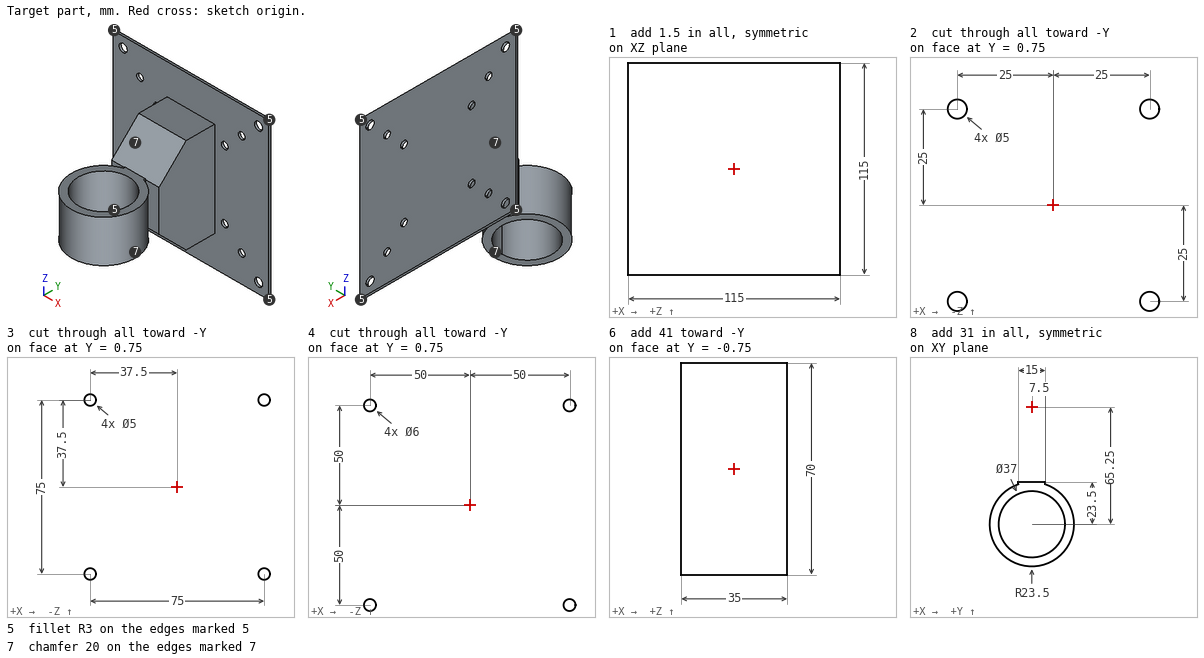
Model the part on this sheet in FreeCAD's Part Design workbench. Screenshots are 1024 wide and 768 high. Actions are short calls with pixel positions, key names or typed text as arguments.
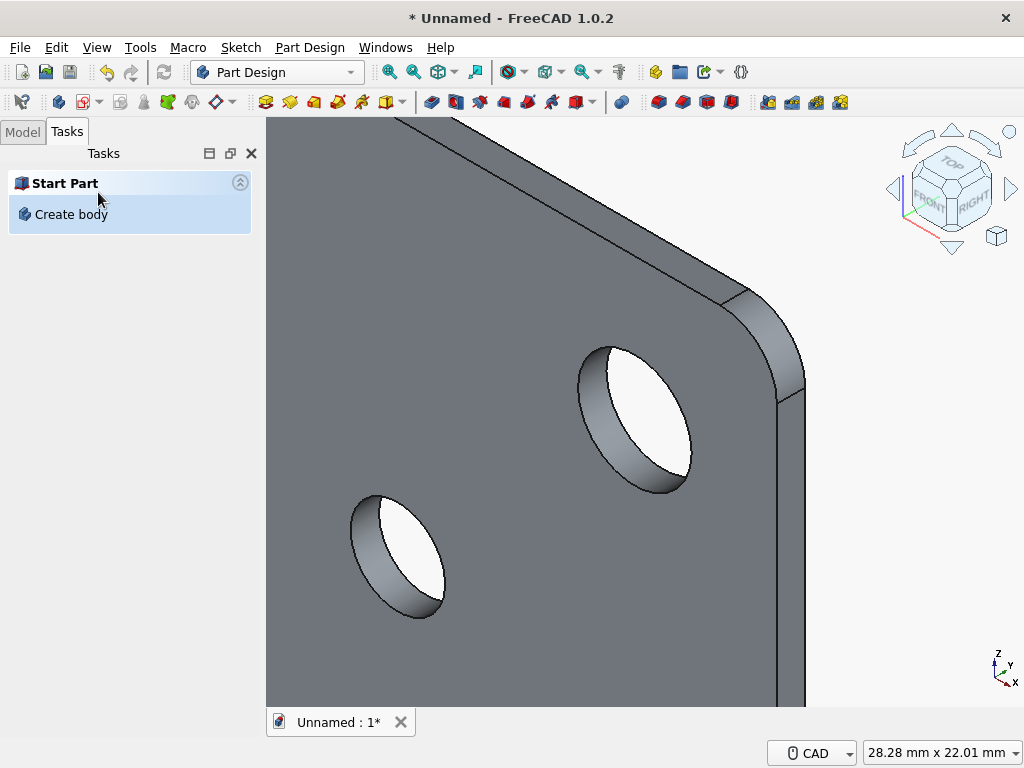
key(v)
key(f)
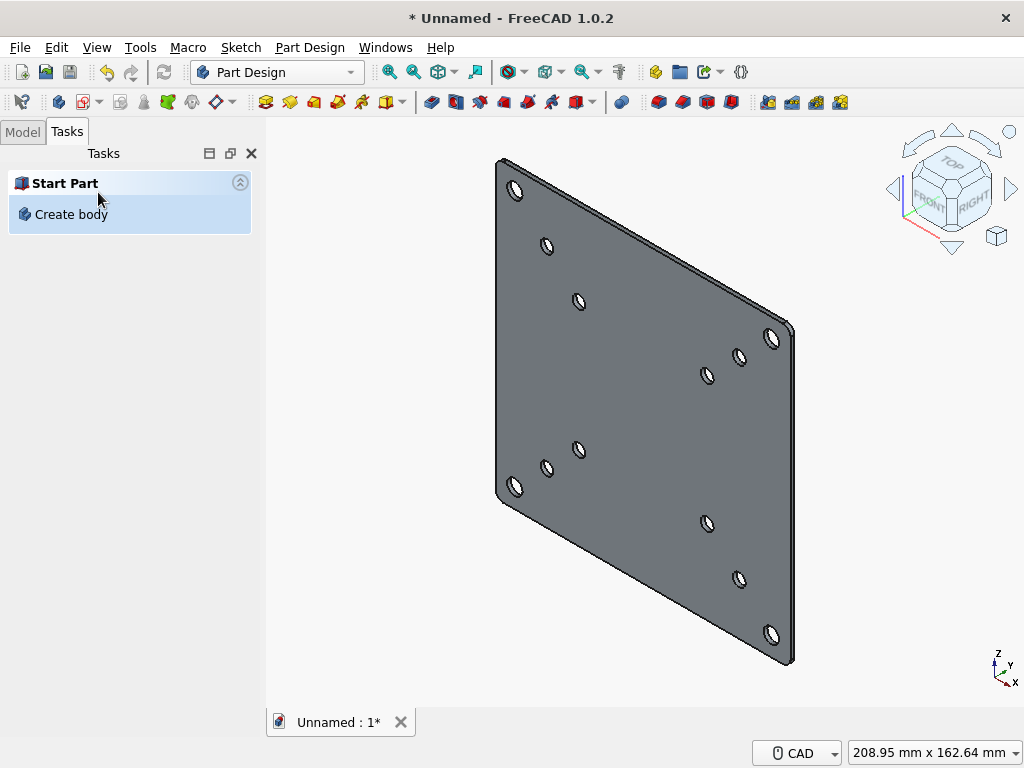
click(643, 412)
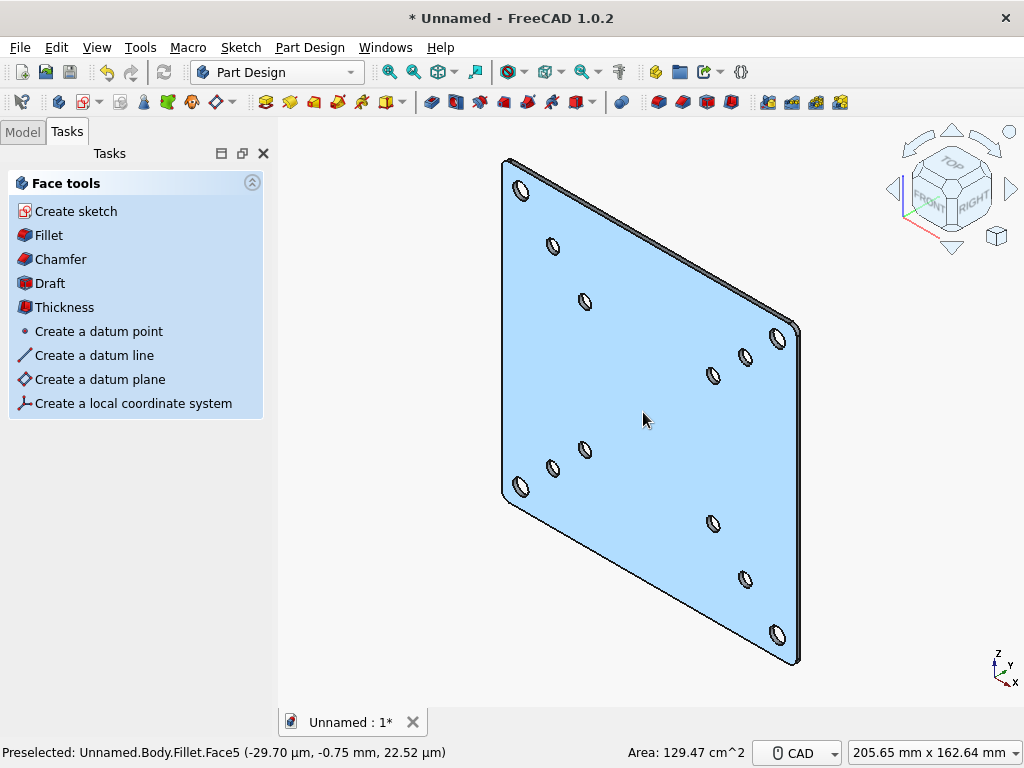
click(84, 102)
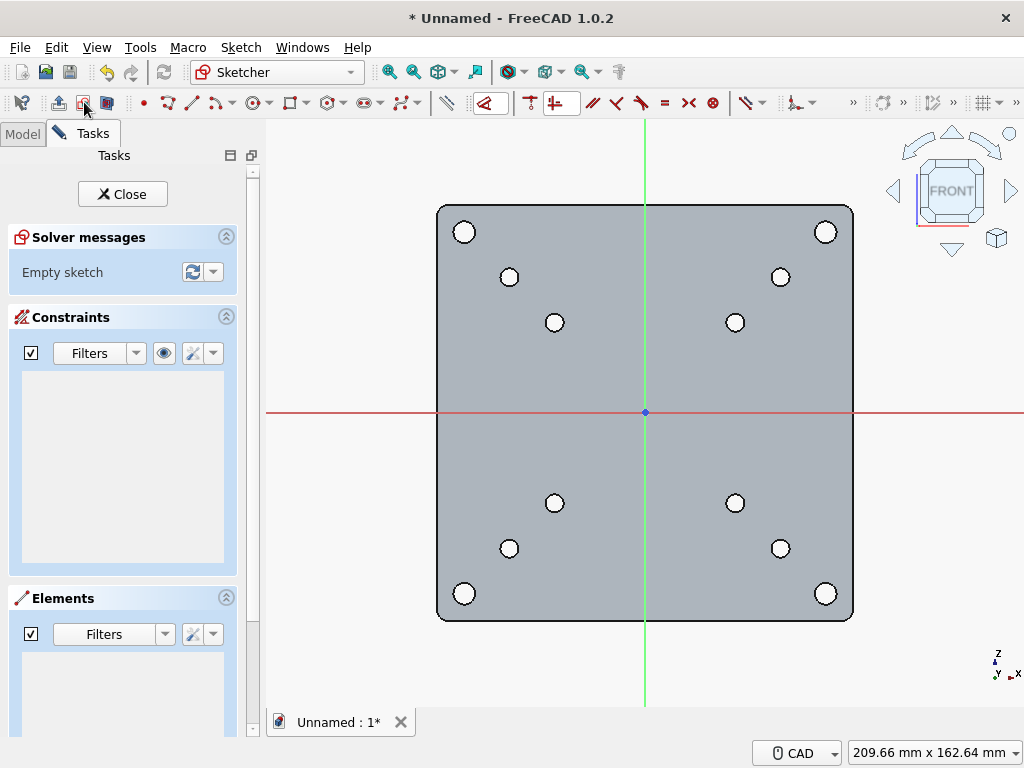
scroll(784, 413, up, 2)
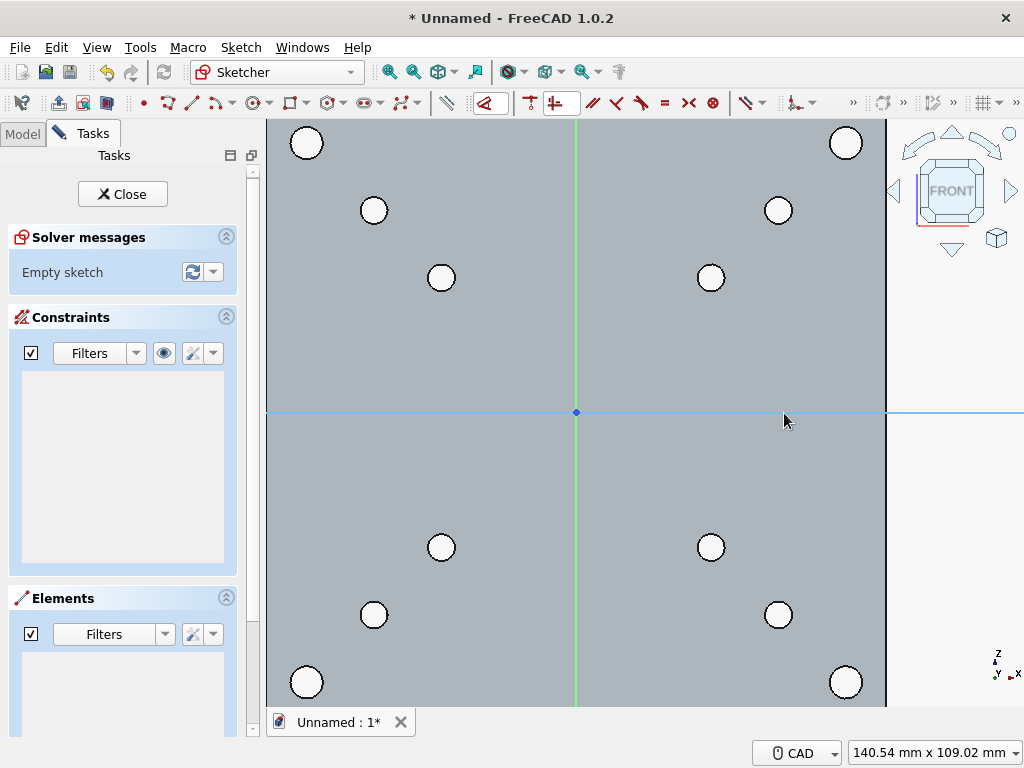
key(g)
key(v)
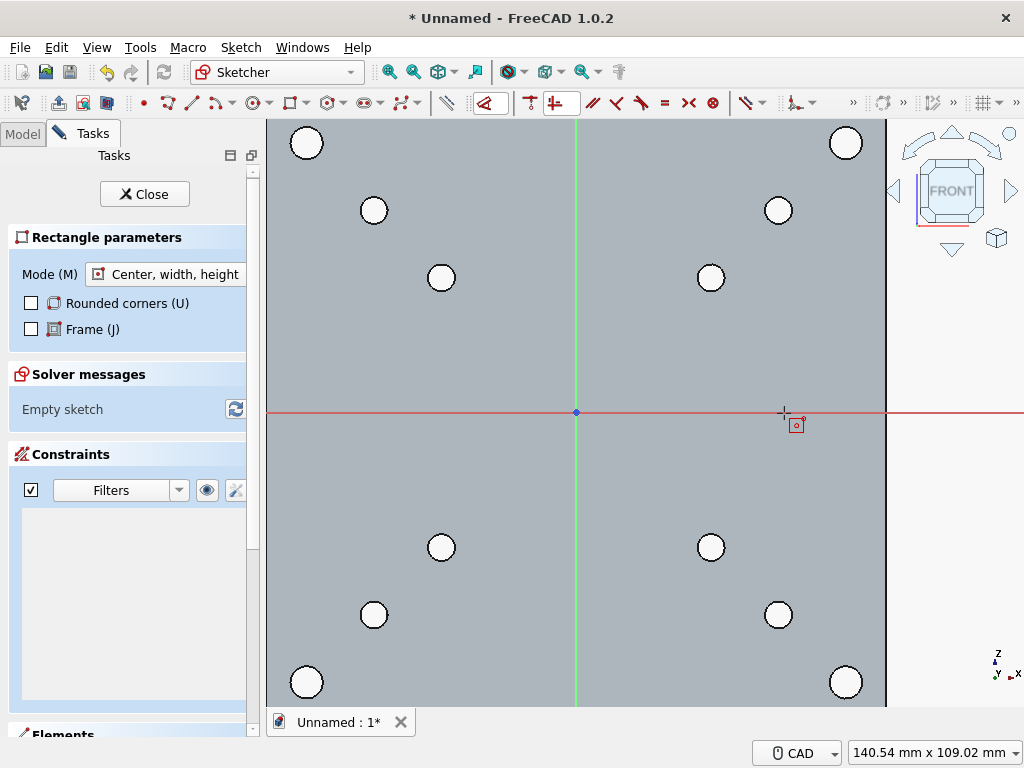
click(576, 413)
click(671, 224)
key(Escape)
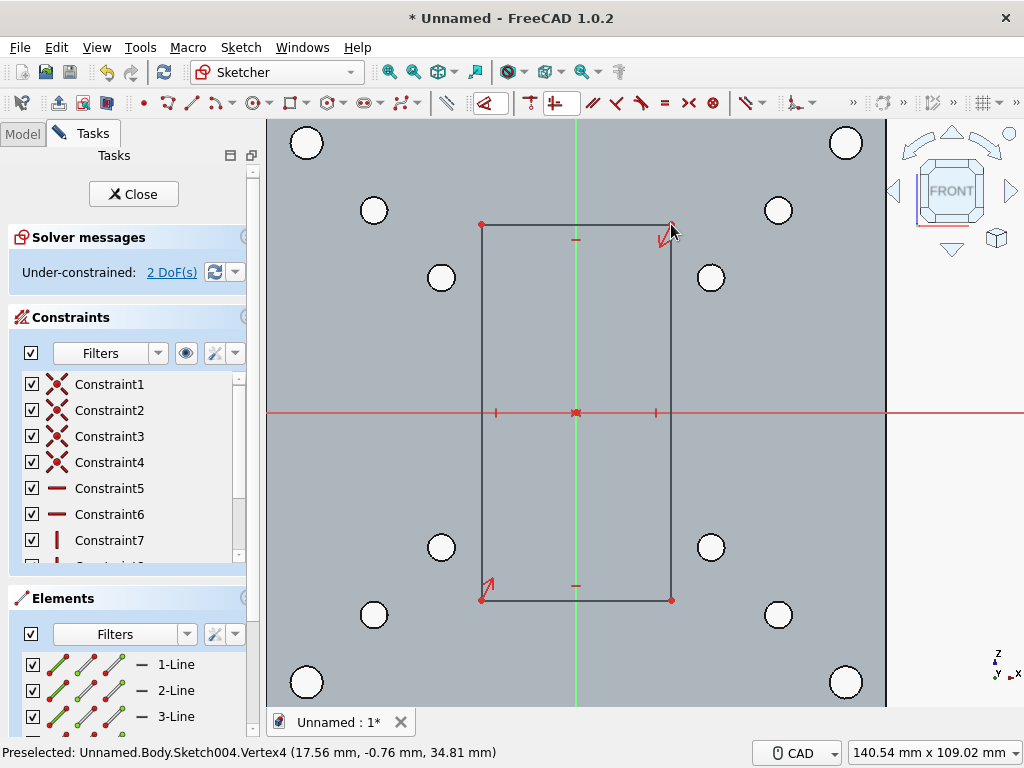
key(d)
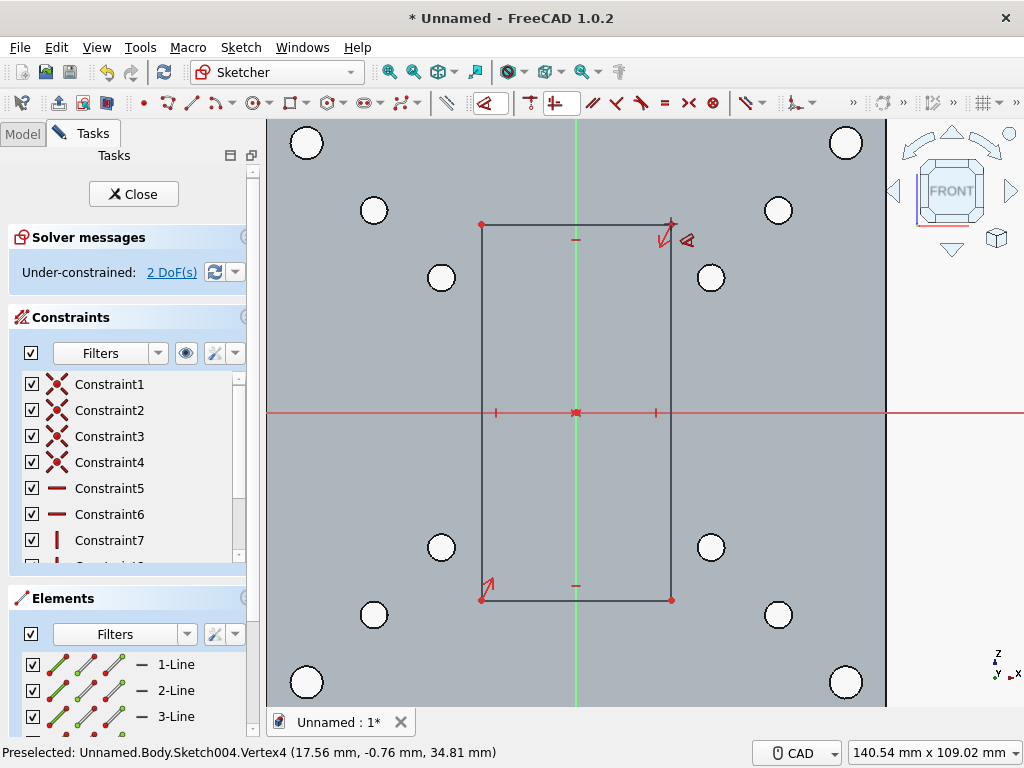
click(538, 601)
click(533, 635)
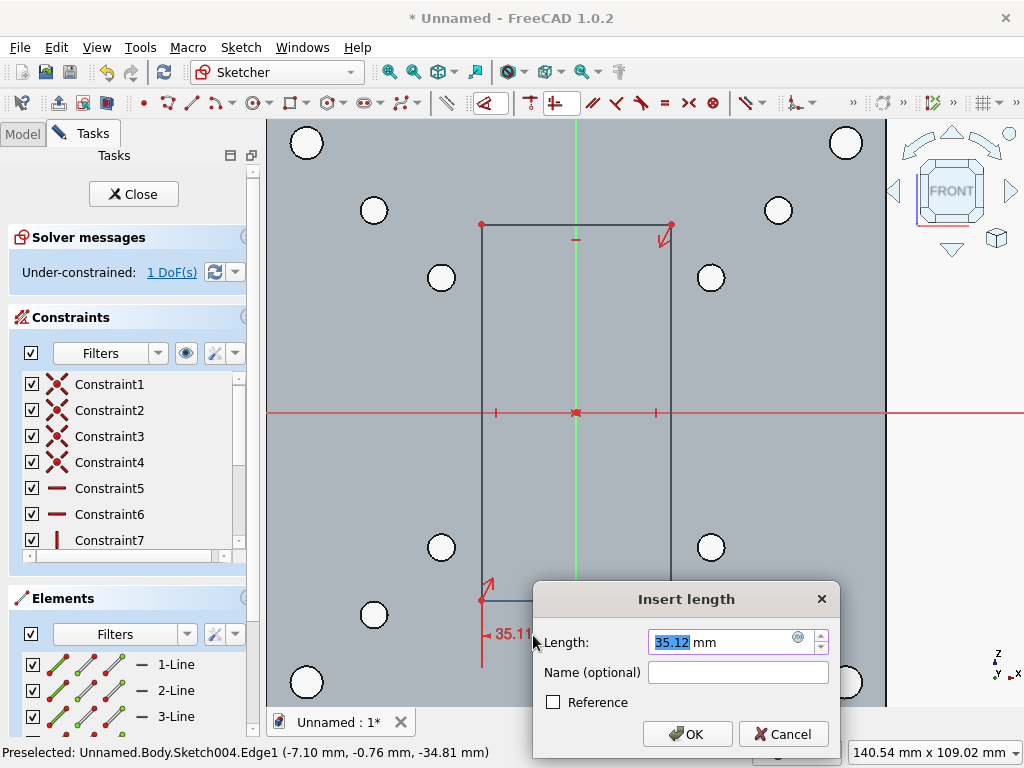
text(35)
key(Return)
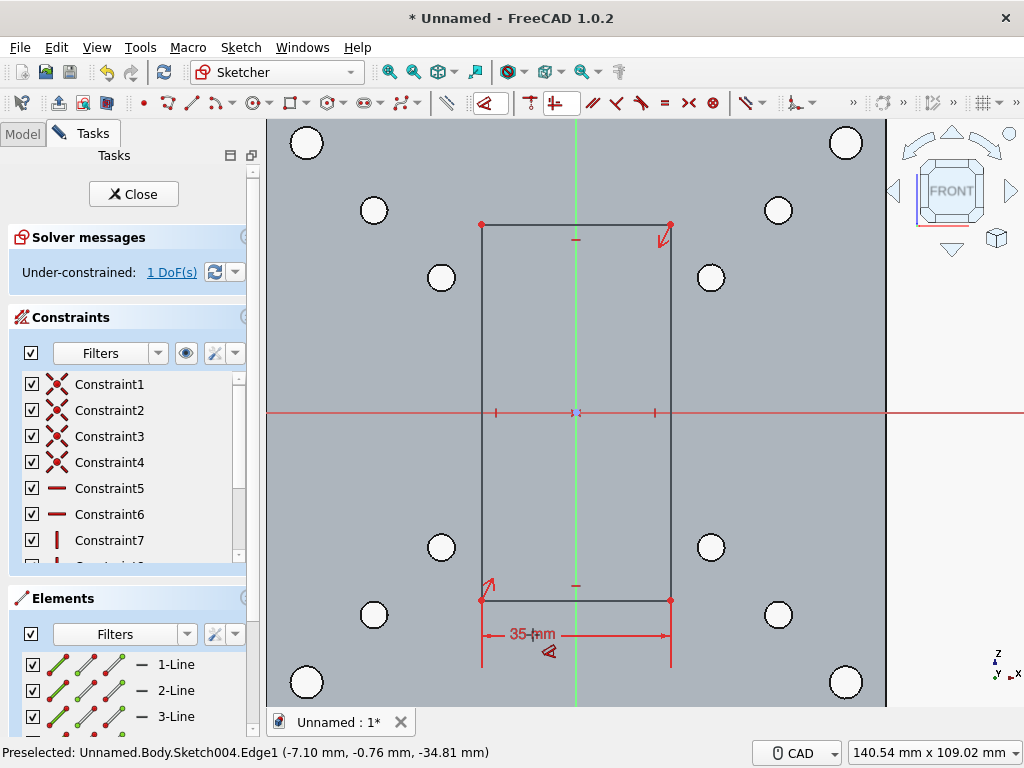
click(671, 488)
click(705, 326)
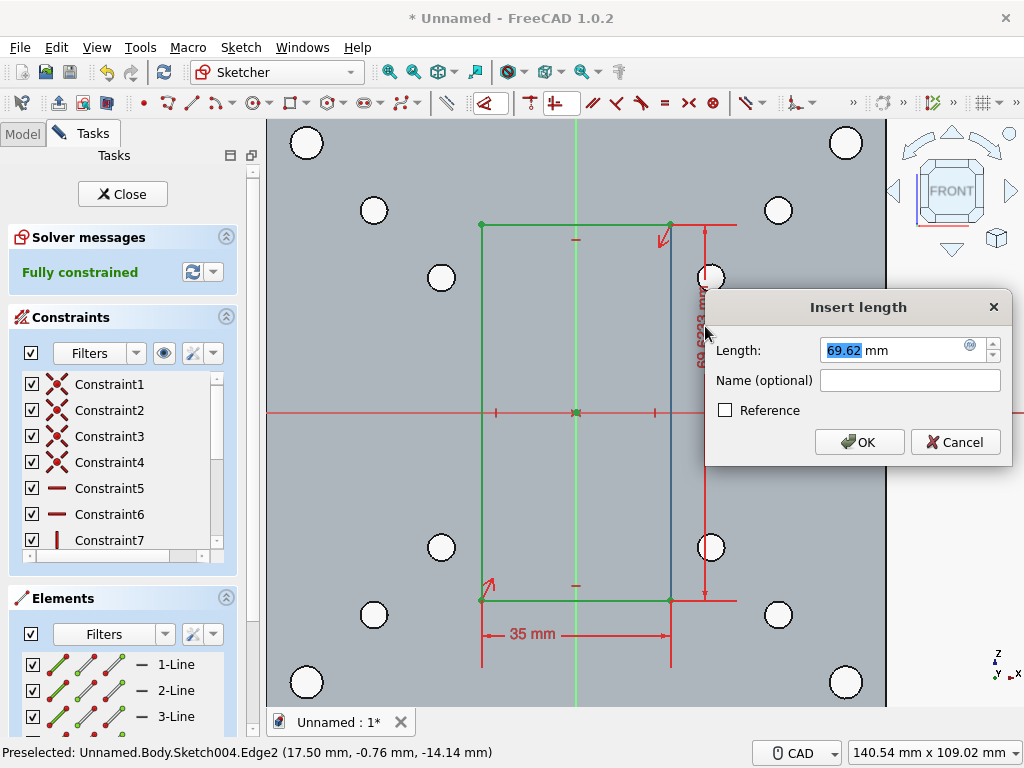
text(70)
key(Return)
key(Escape)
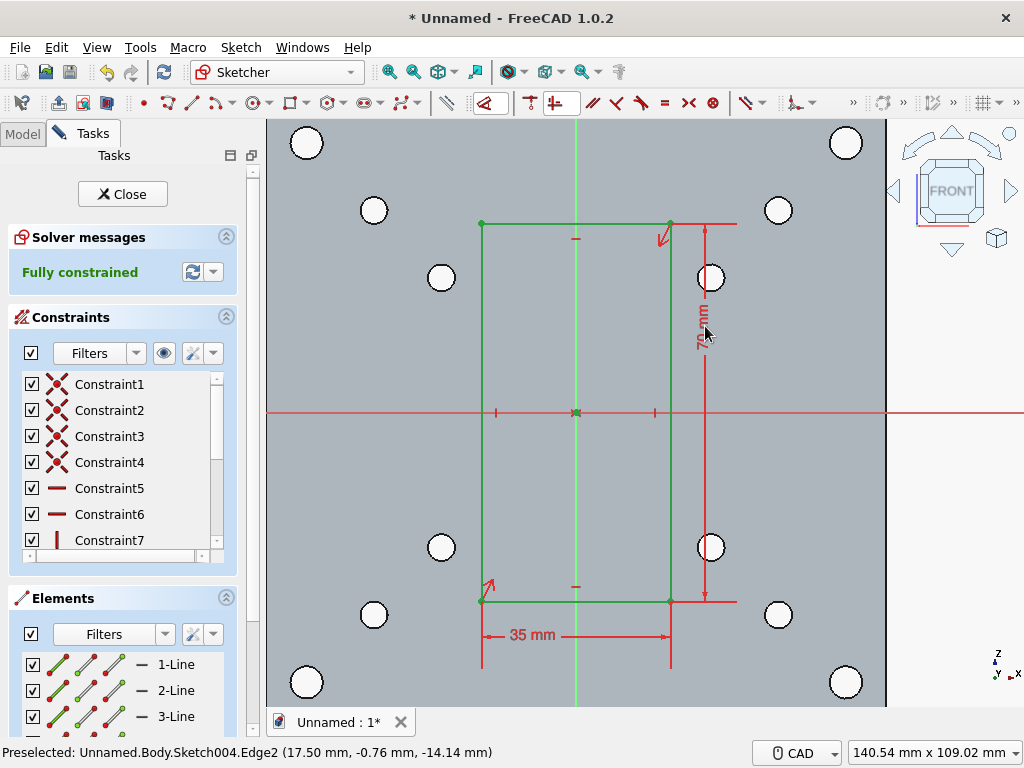
click(123, 194)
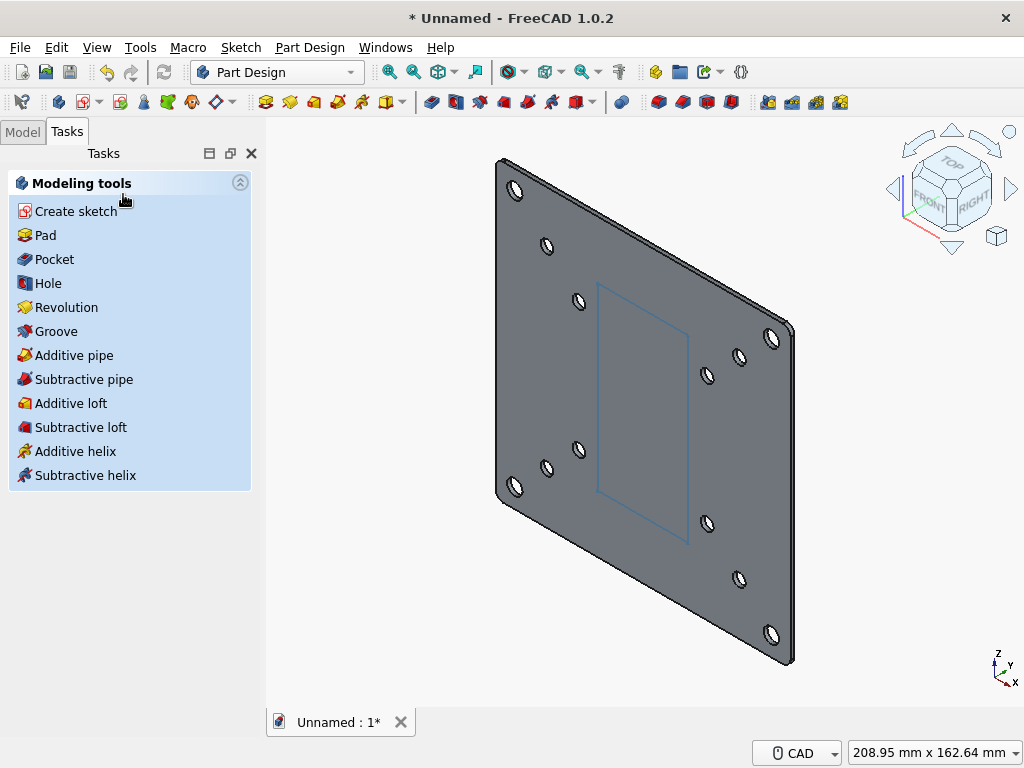
click(266, 102)